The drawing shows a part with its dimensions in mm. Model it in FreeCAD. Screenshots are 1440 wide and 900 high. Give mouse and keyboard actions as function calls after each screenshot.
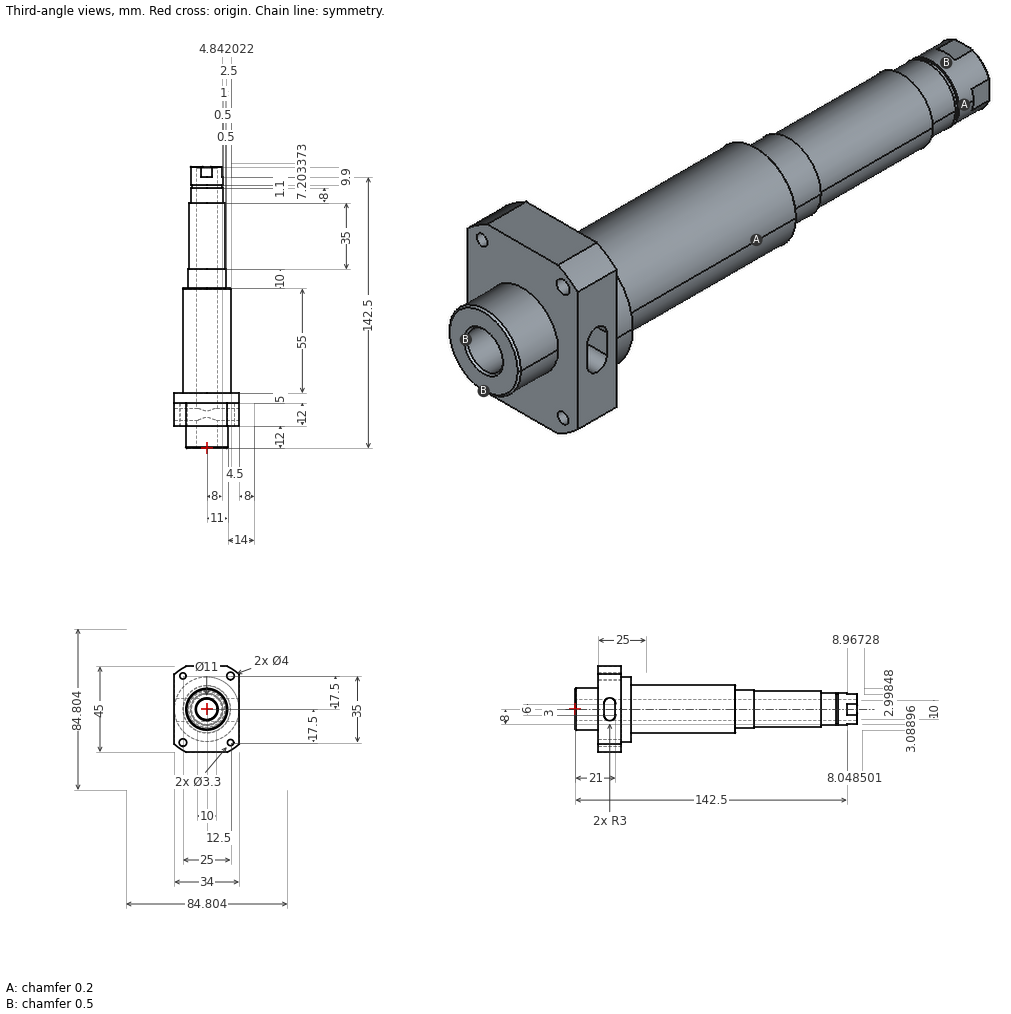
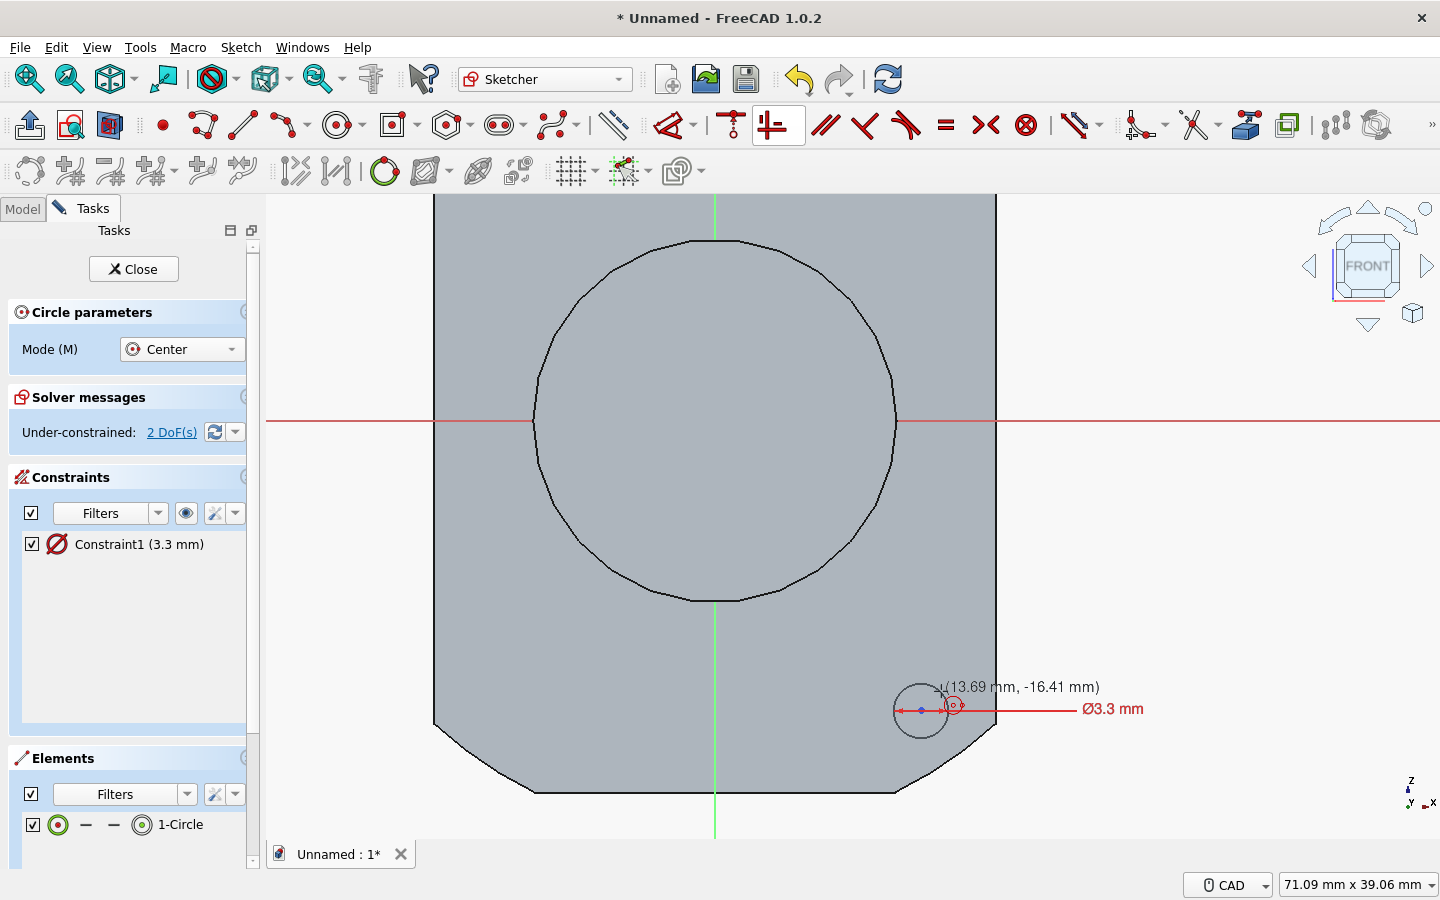
scroll(926, 711, down, 2)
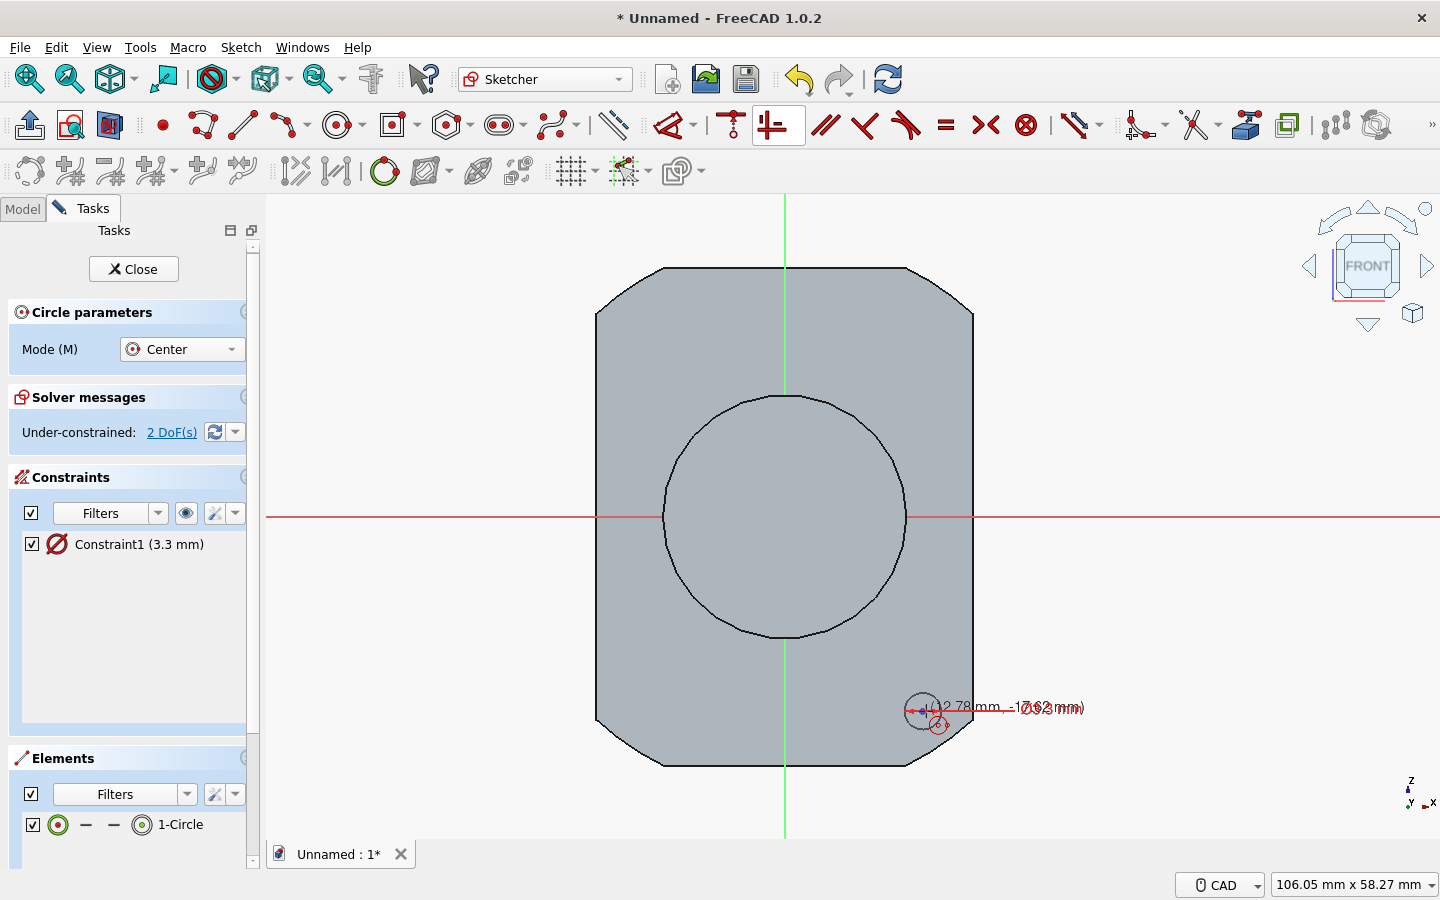
scroll(646, 323, up, 2)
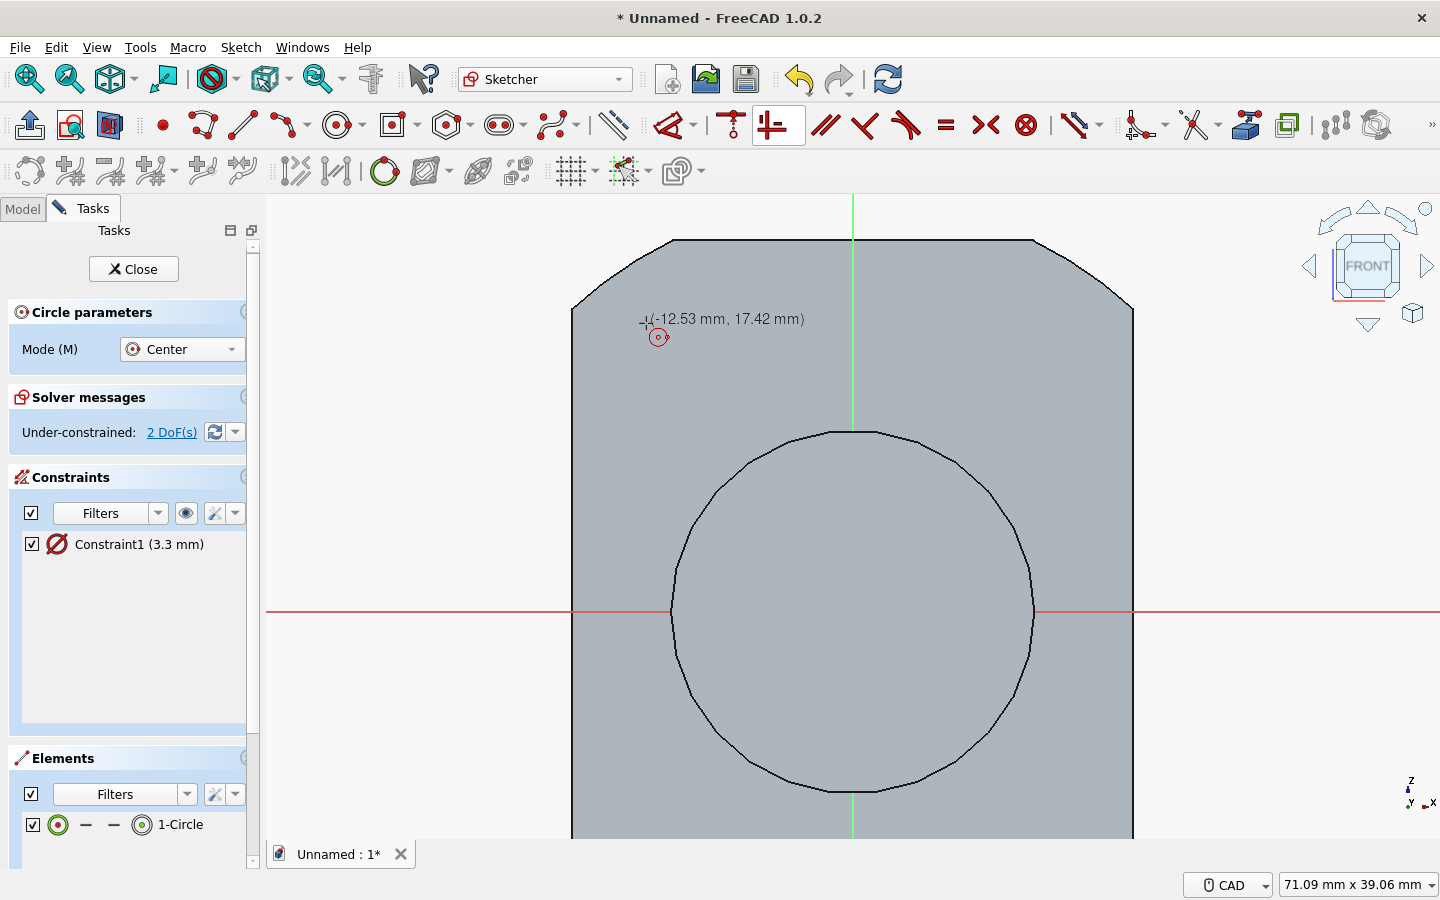
click(646, 323)
move(666, 304)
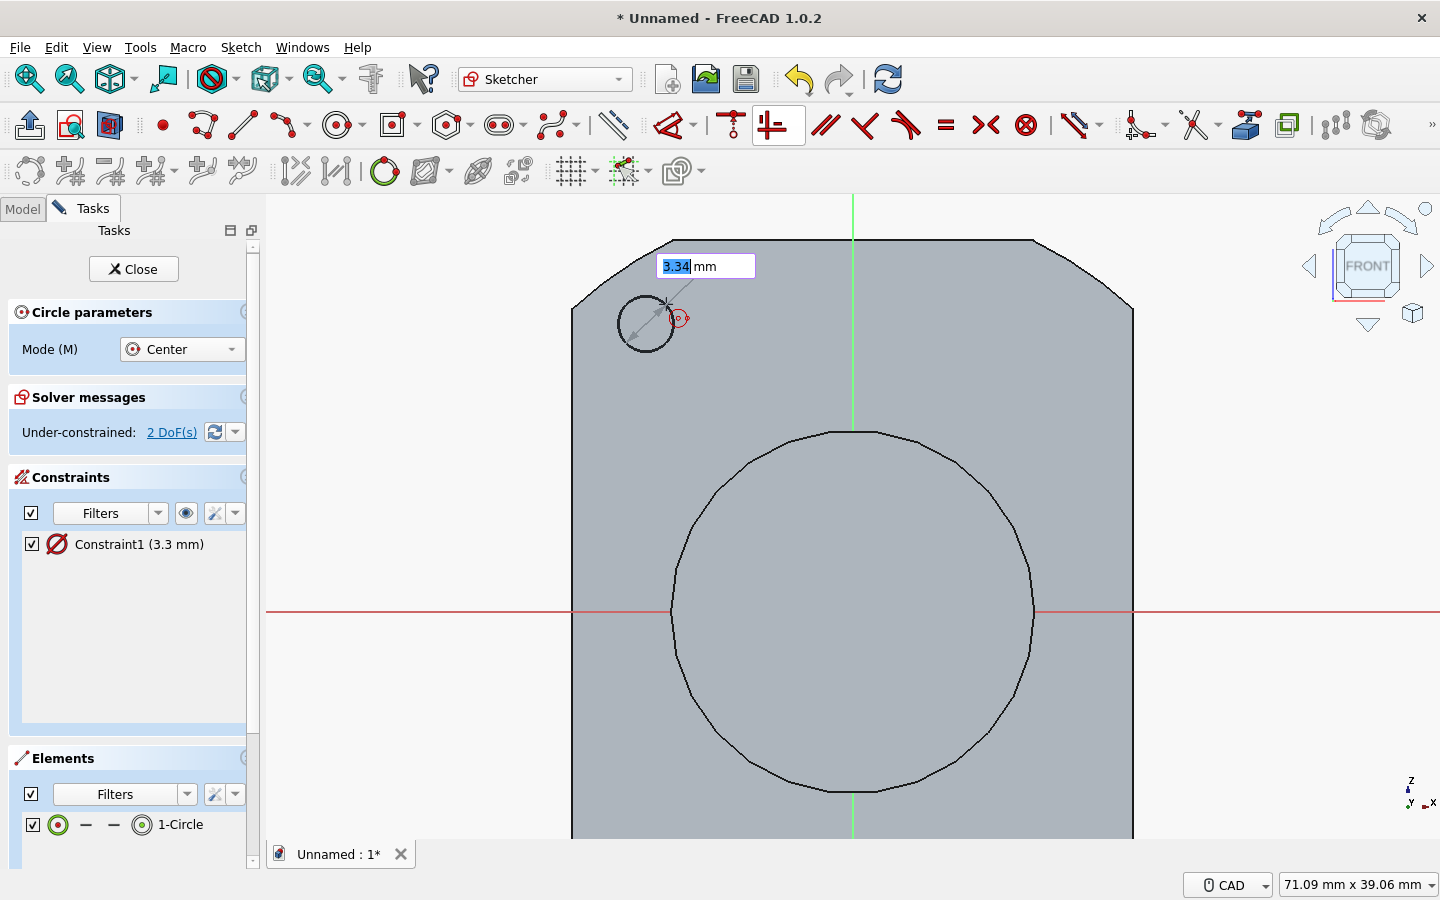
text(3.3)
key(Return)
key(Escape)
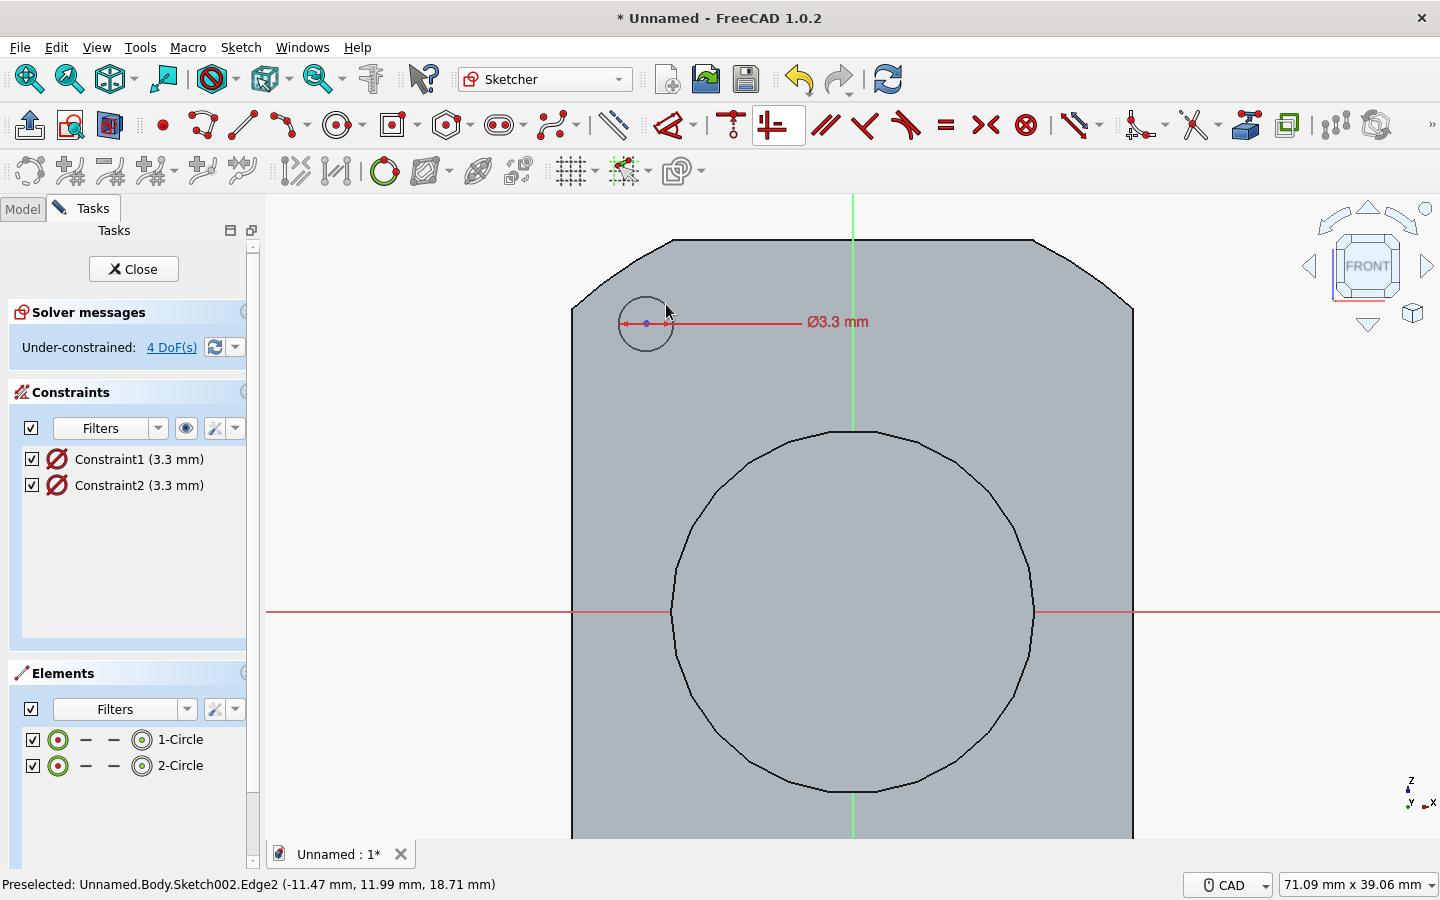
click(668, 126)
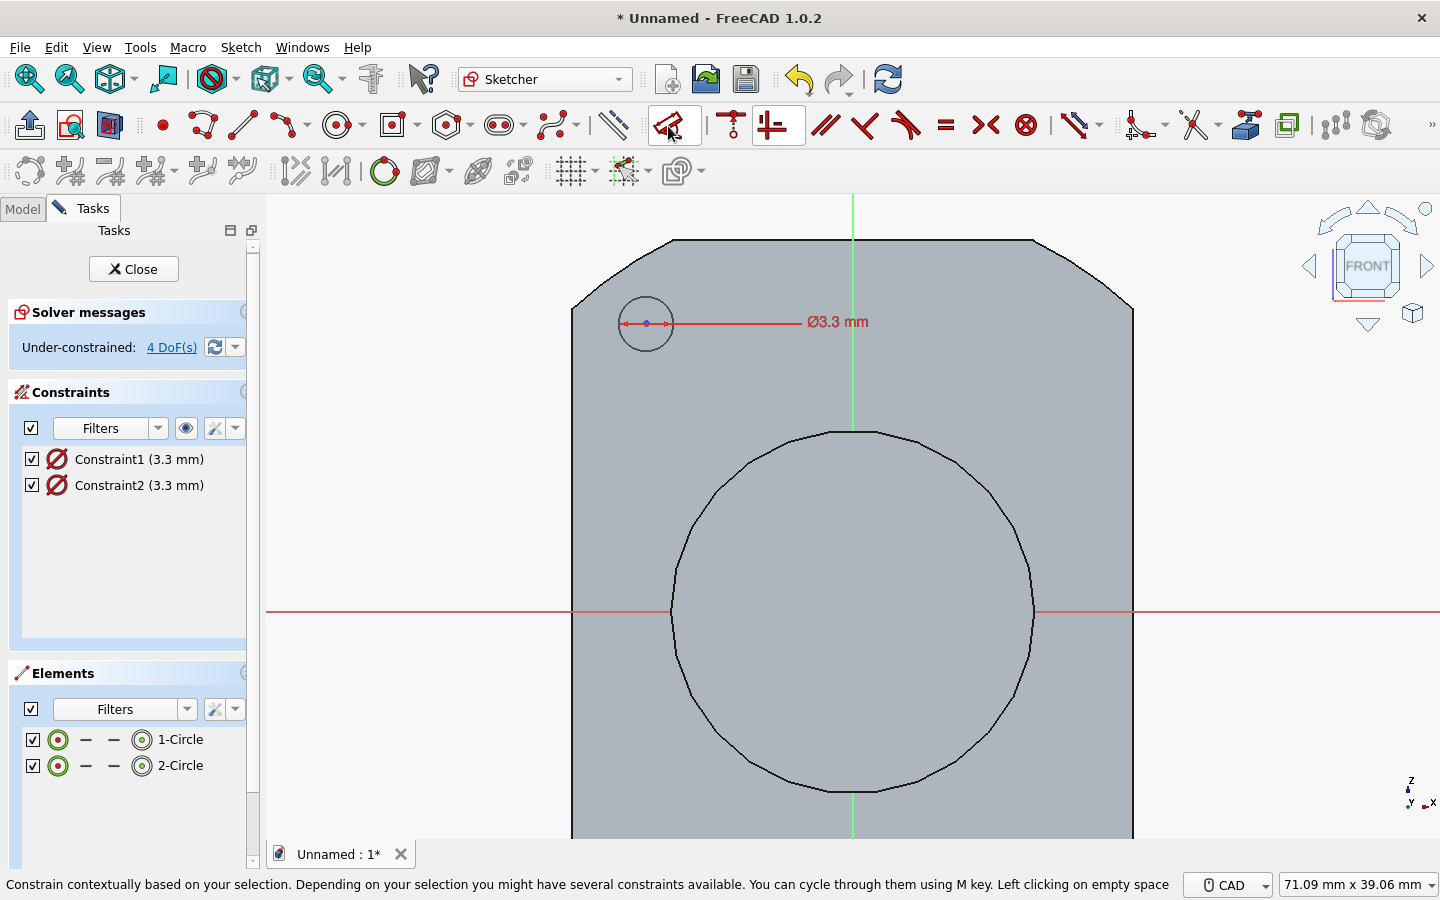
scroll(646, 322, down, 2)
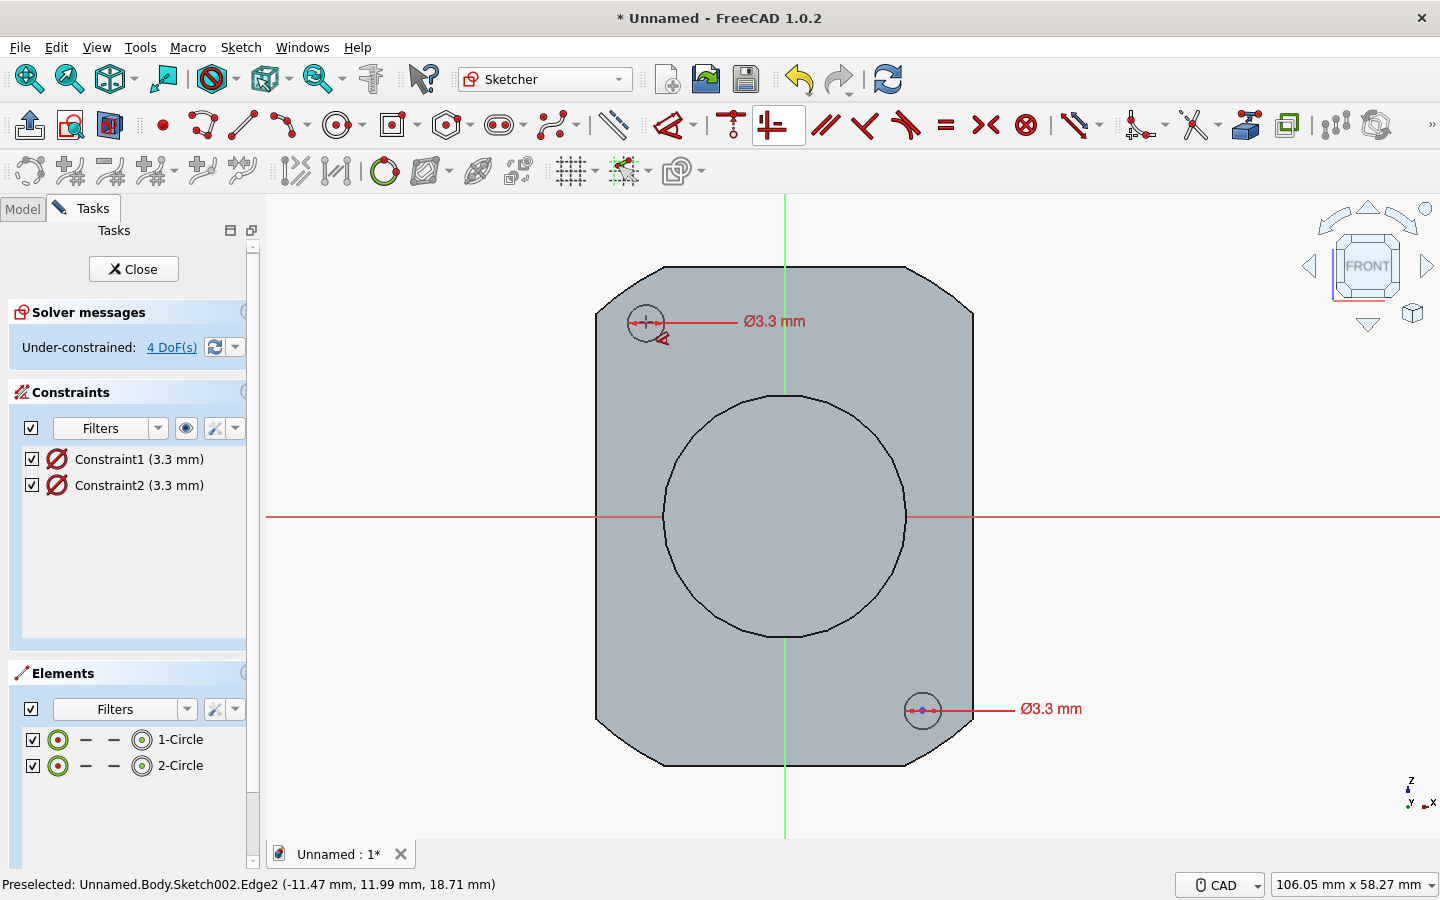
click(923, 711)